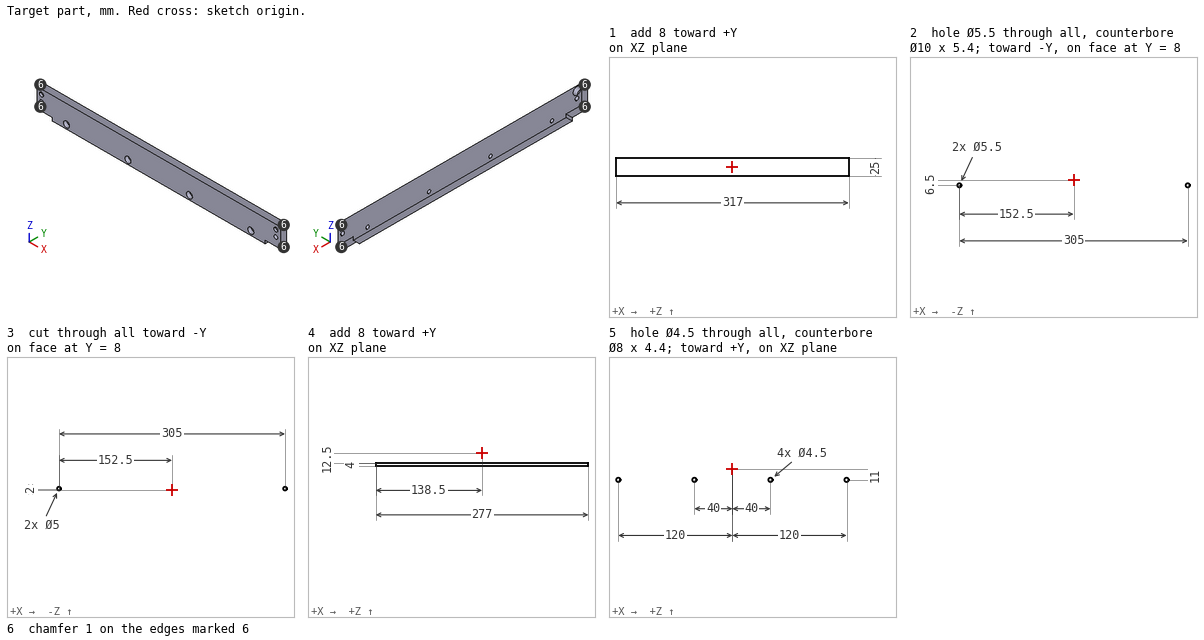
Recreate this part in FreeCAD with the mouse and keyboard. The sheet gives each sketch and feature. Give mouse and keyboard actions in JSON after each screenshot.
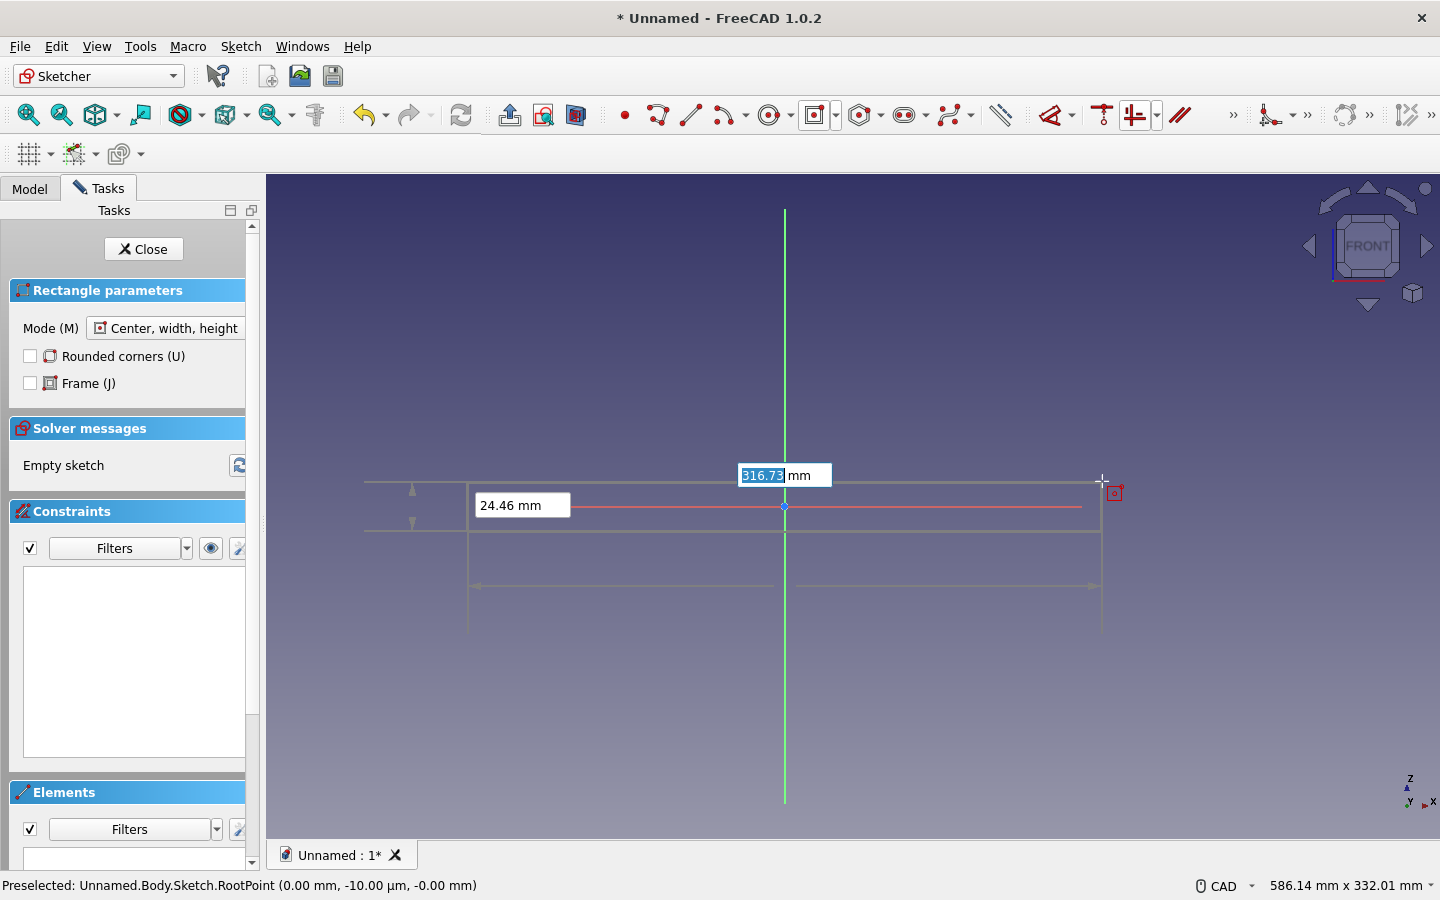
{"action": "type", "text": "317"}
{"action": "key", "text": "Tab"}
{"action": "type", "text": "25"}
{"action": "key", "text": "Return"}
{"action": "key", "text": "Escape"}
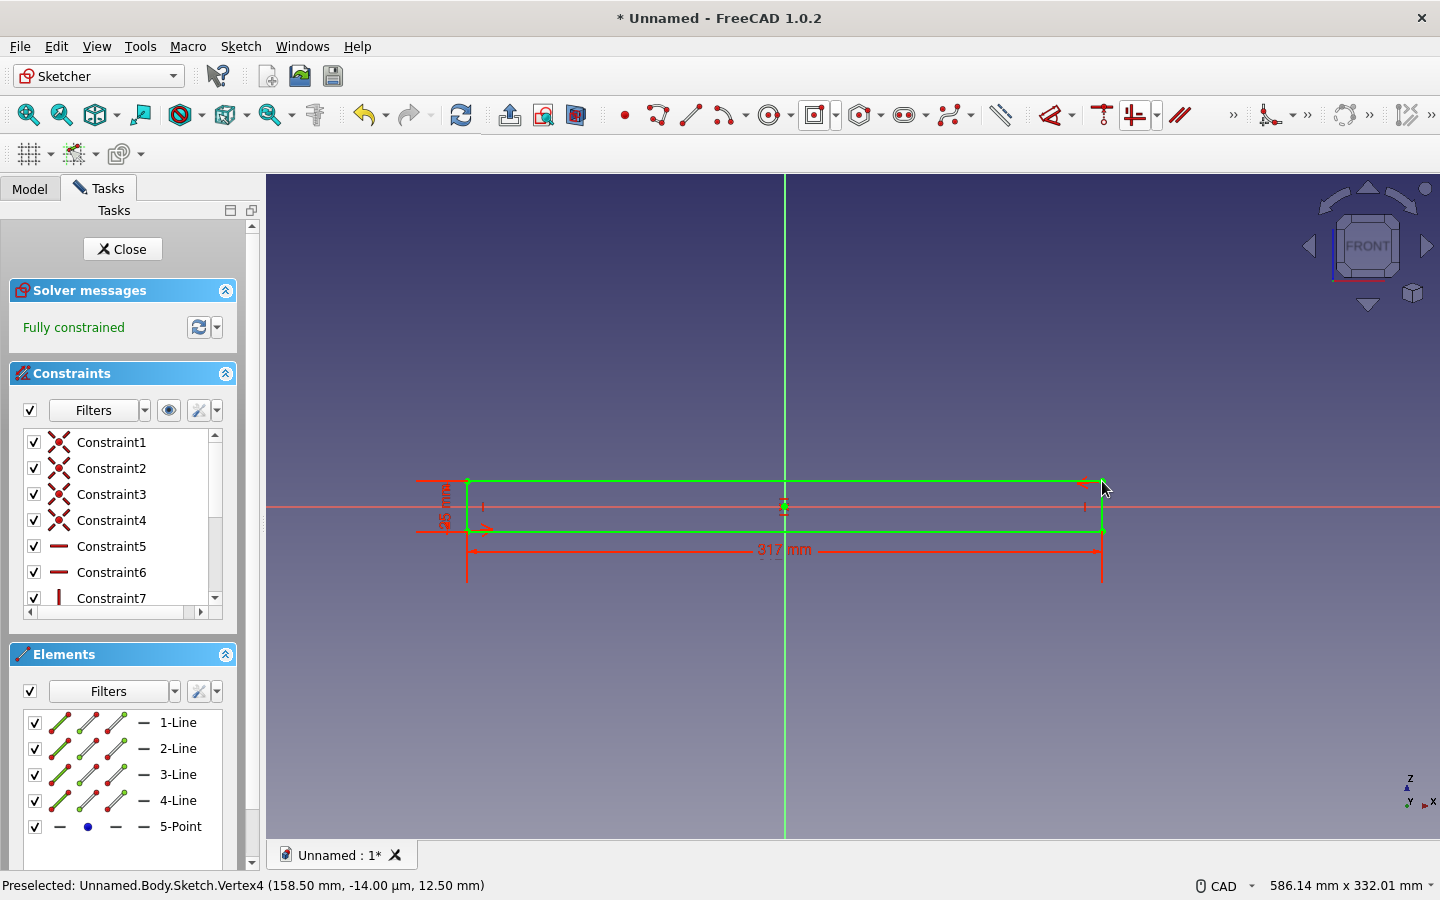
{"action": "left_click", "coordinate": [123, 249]}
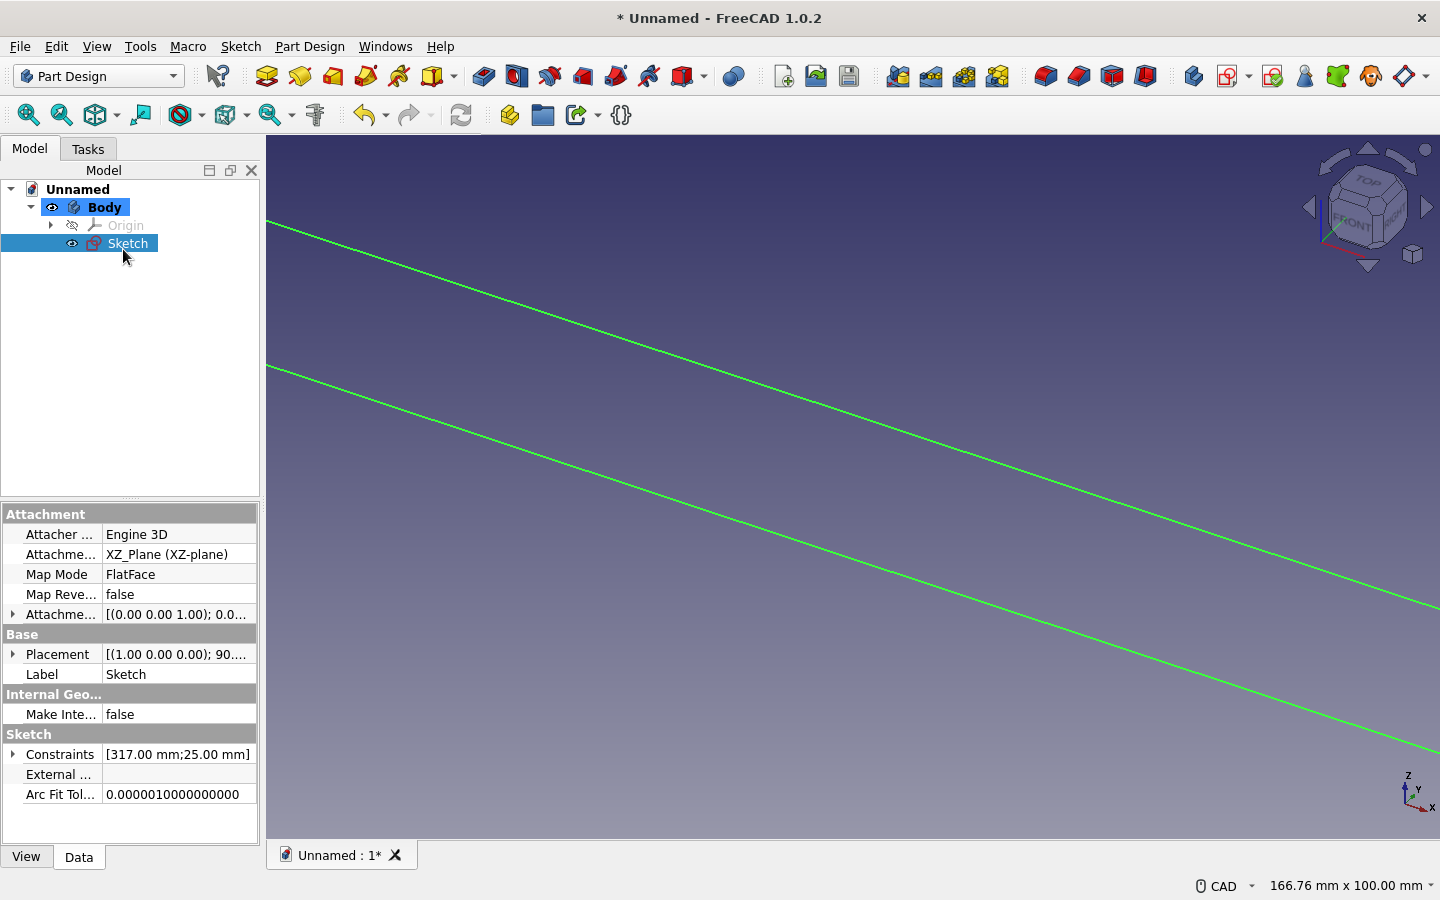
{"action": "left_click", "coordinate": [267, 76]}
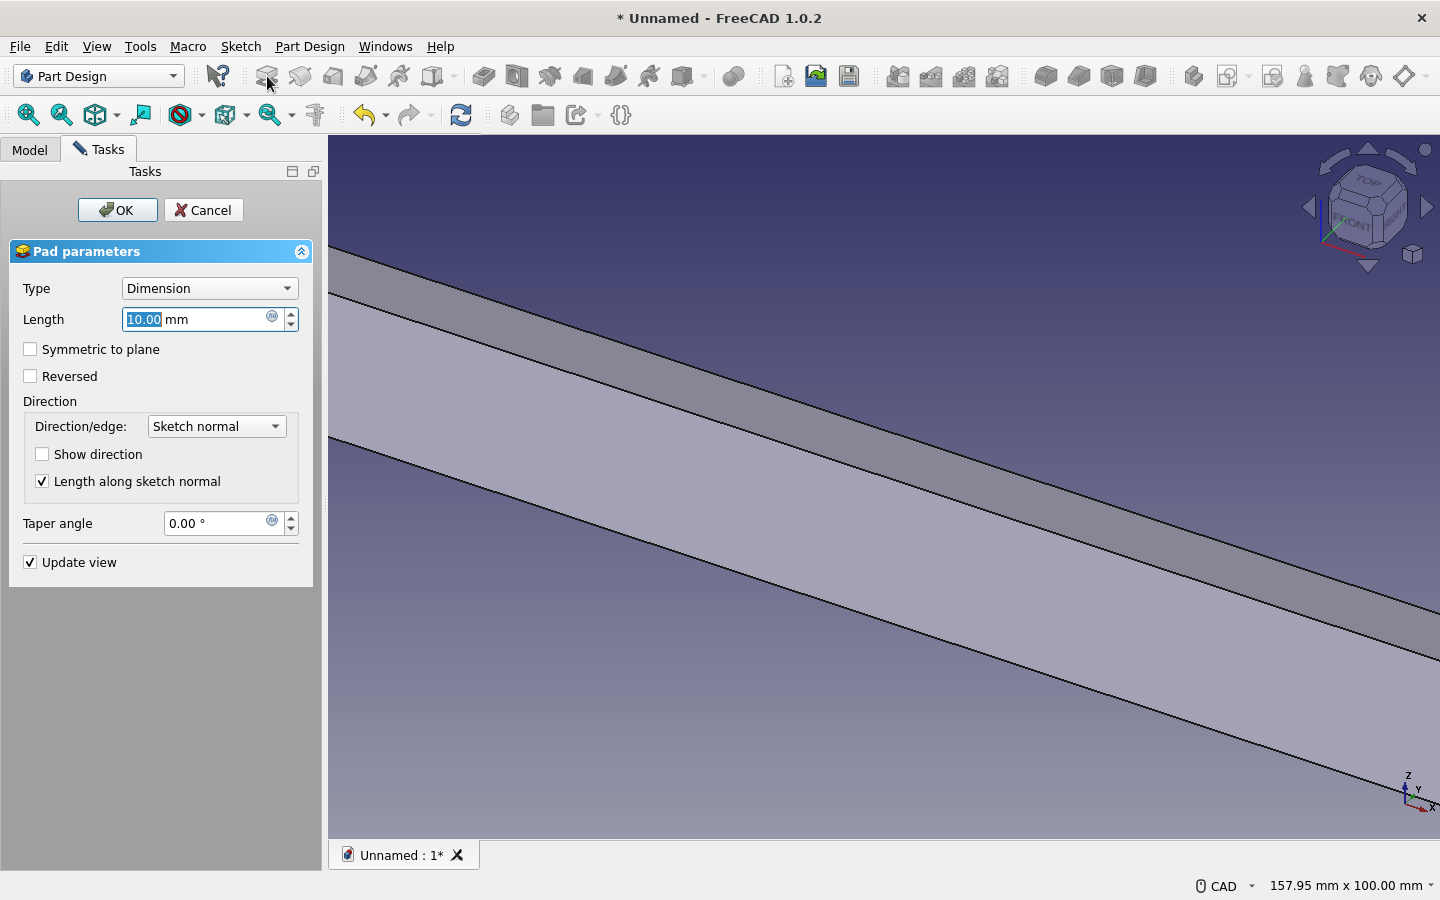
{"action": "type", "text": "8"}
{"action": "key", "text": "Tab"}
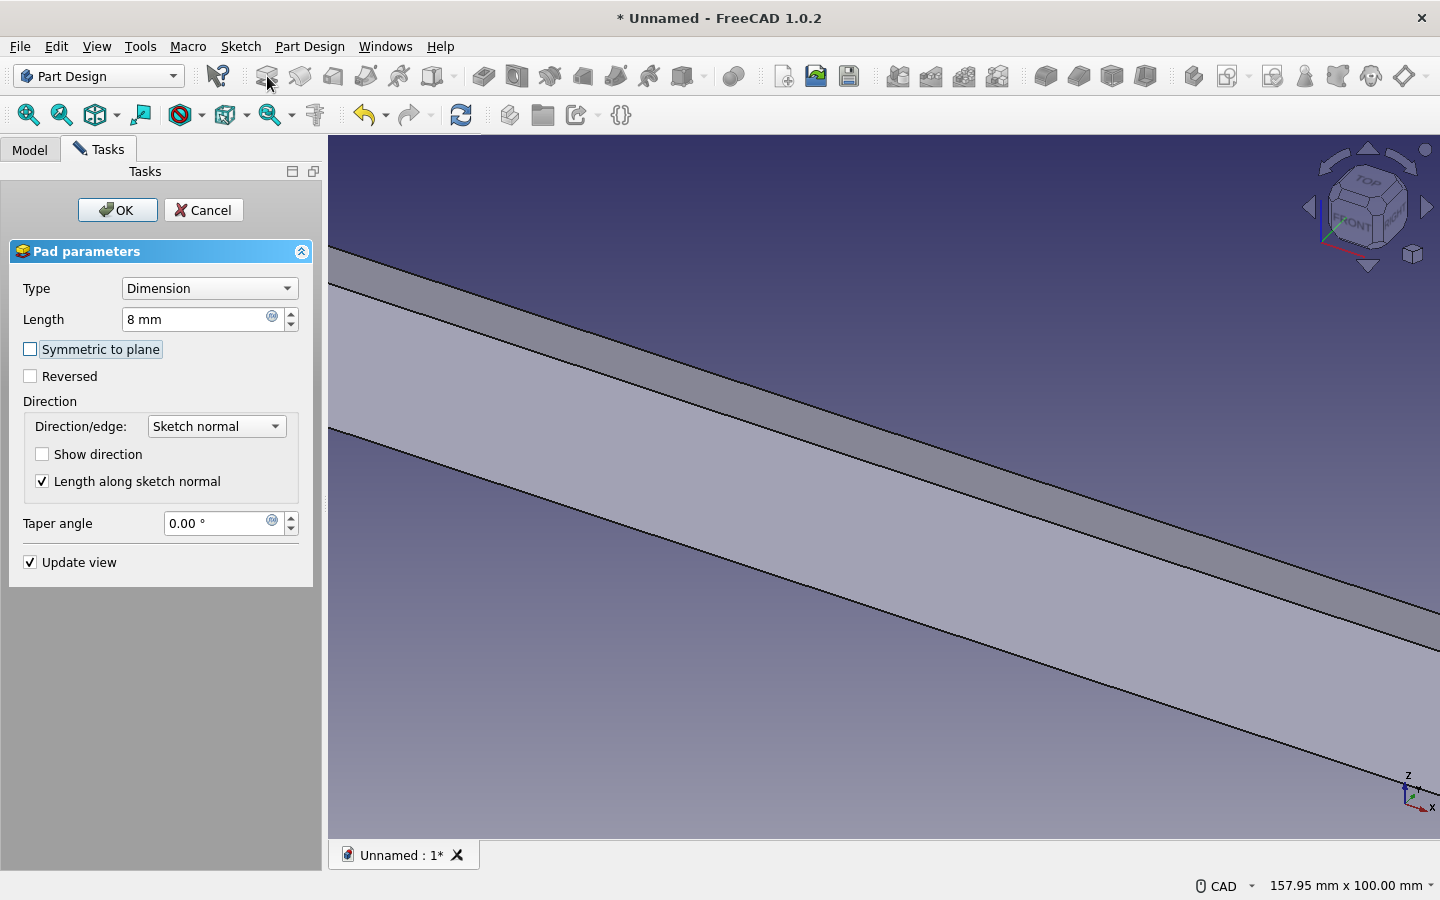
{"action": "left_click", "coordinate": [31, 376]}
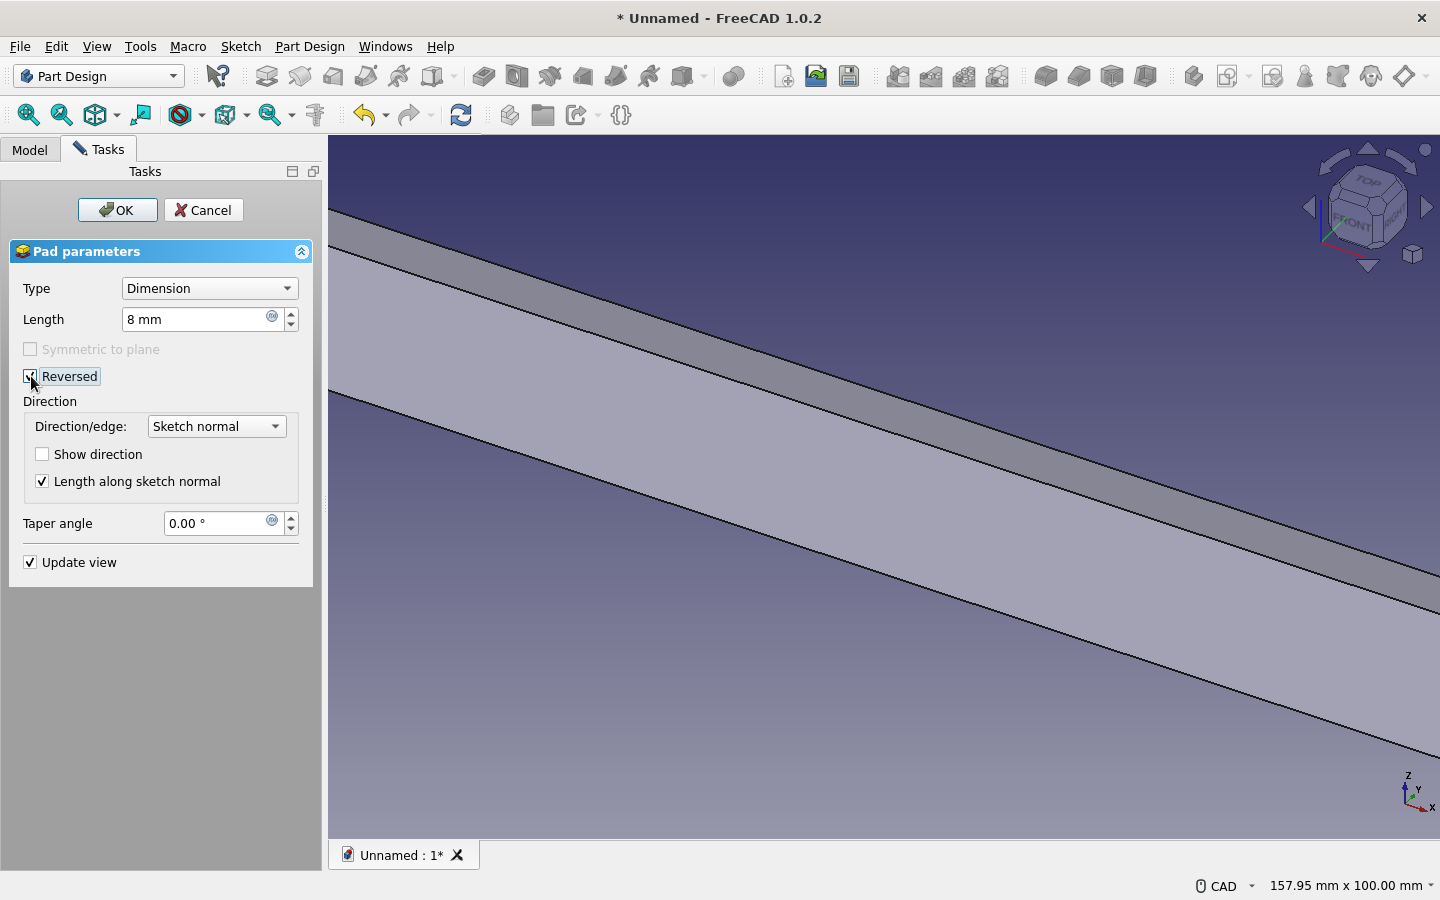
{"action": "left_click", "coordinate": [118, 210]}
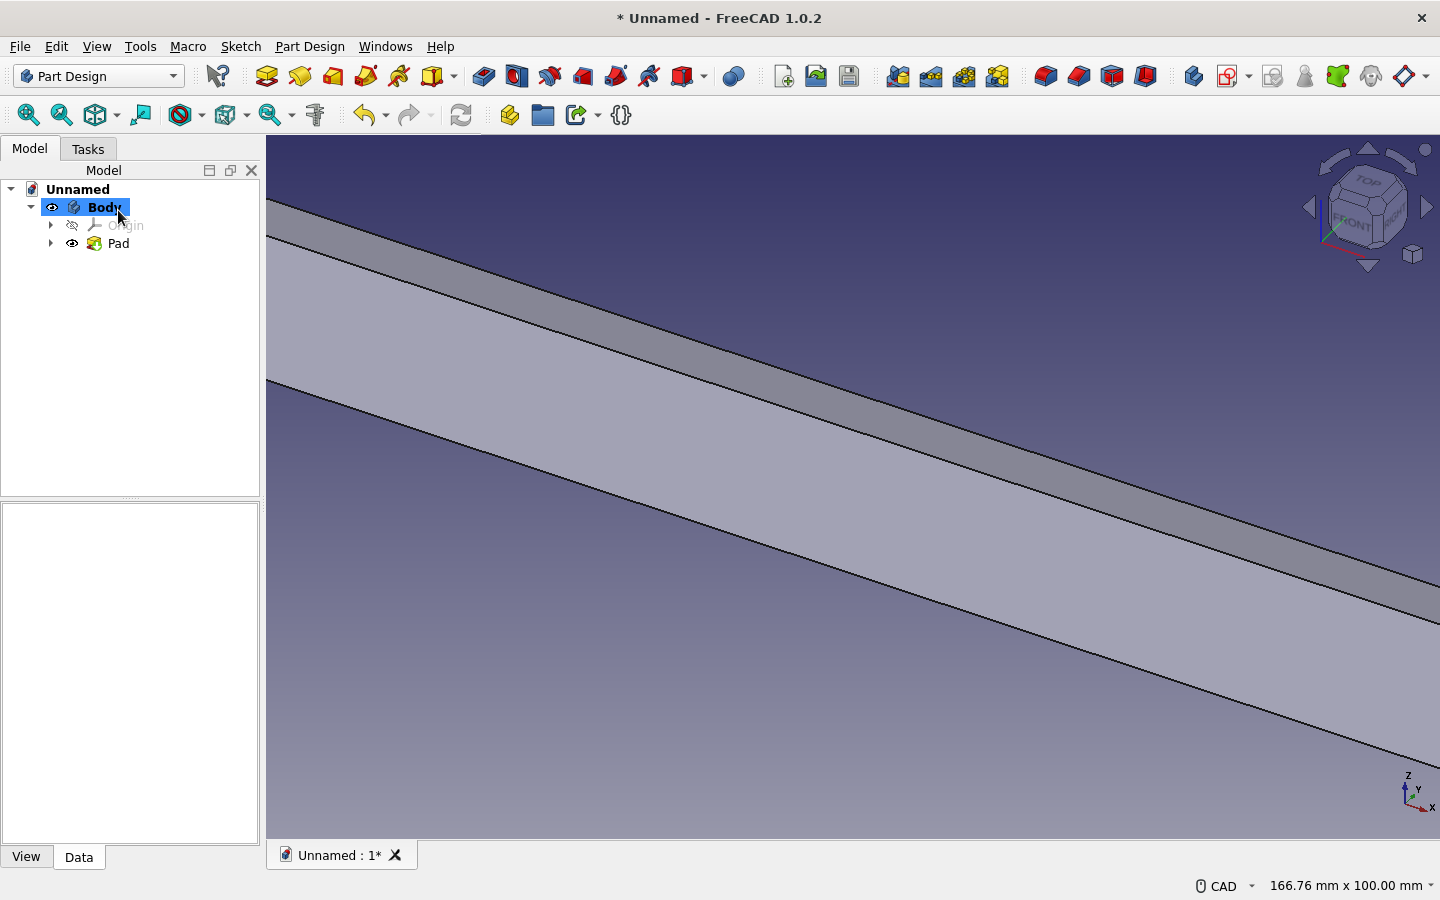
{"action": "left_click", "coordinate": [29, 116]}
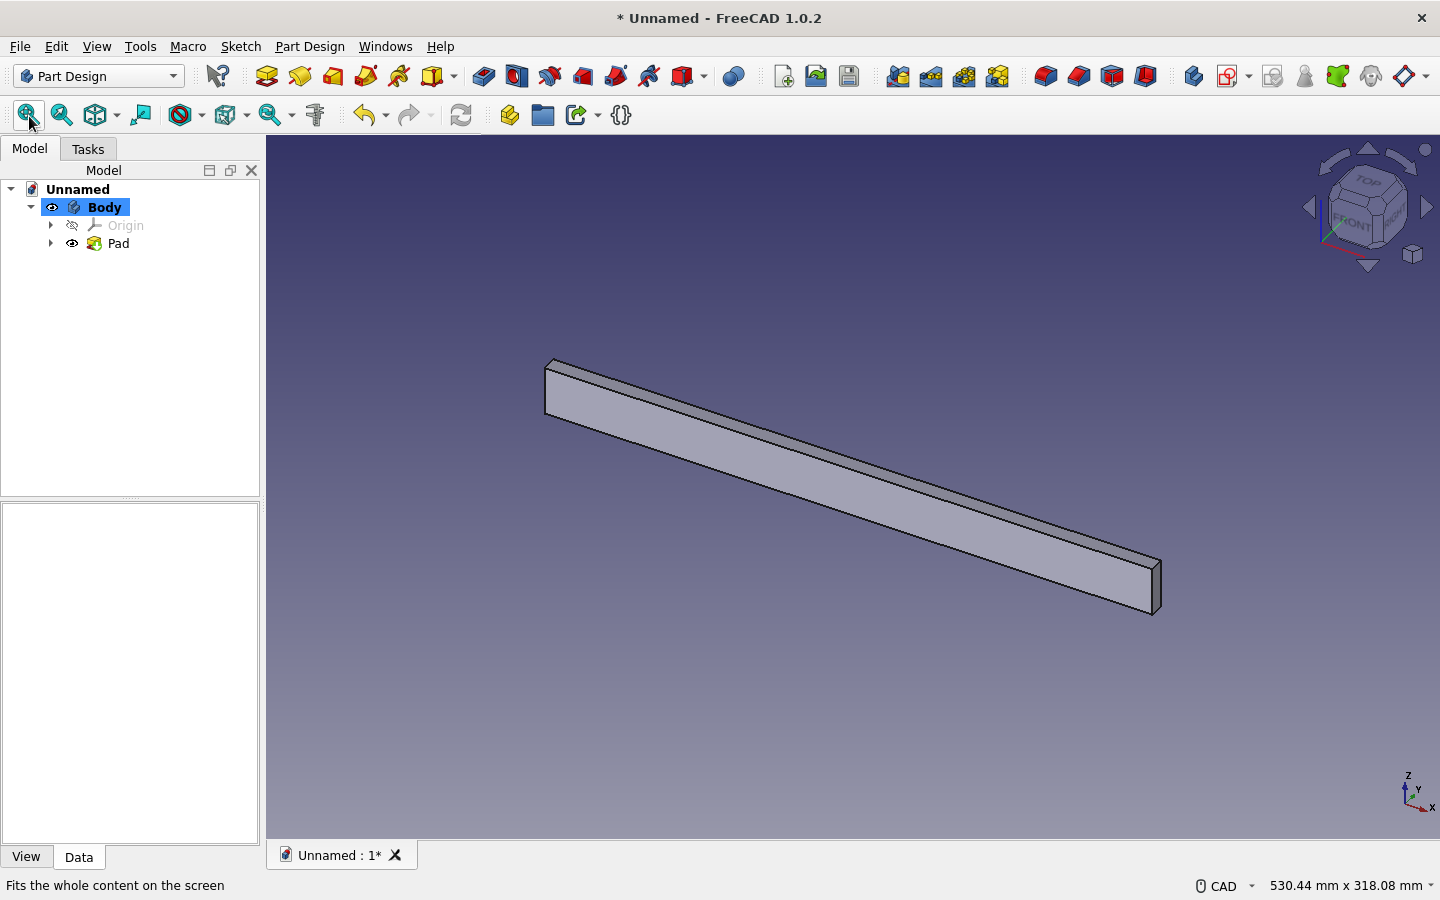
{"action": "key", "text": "4"}